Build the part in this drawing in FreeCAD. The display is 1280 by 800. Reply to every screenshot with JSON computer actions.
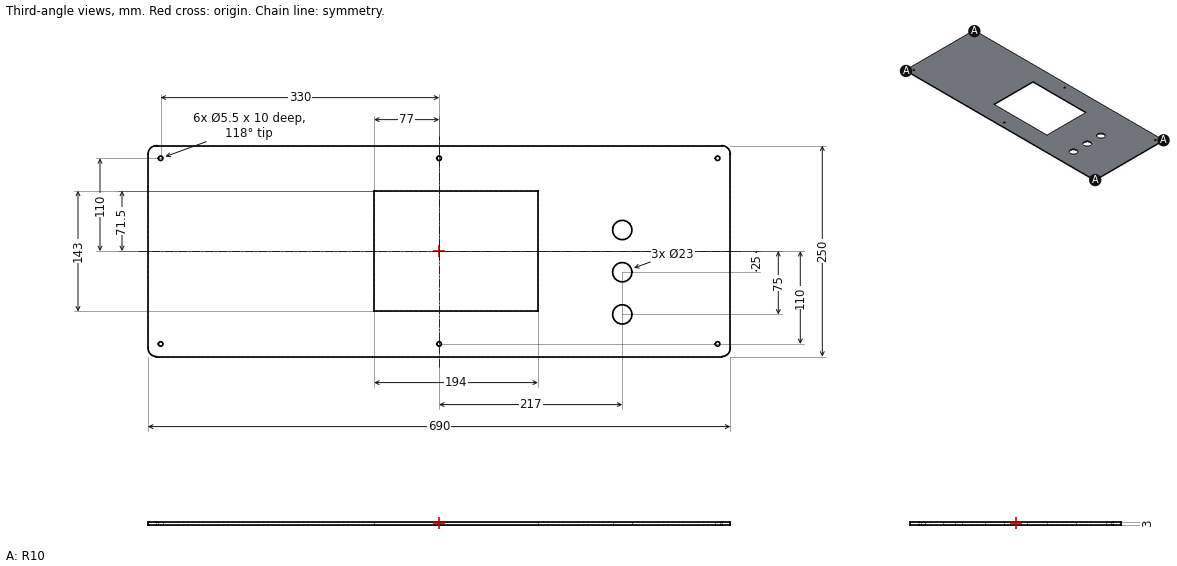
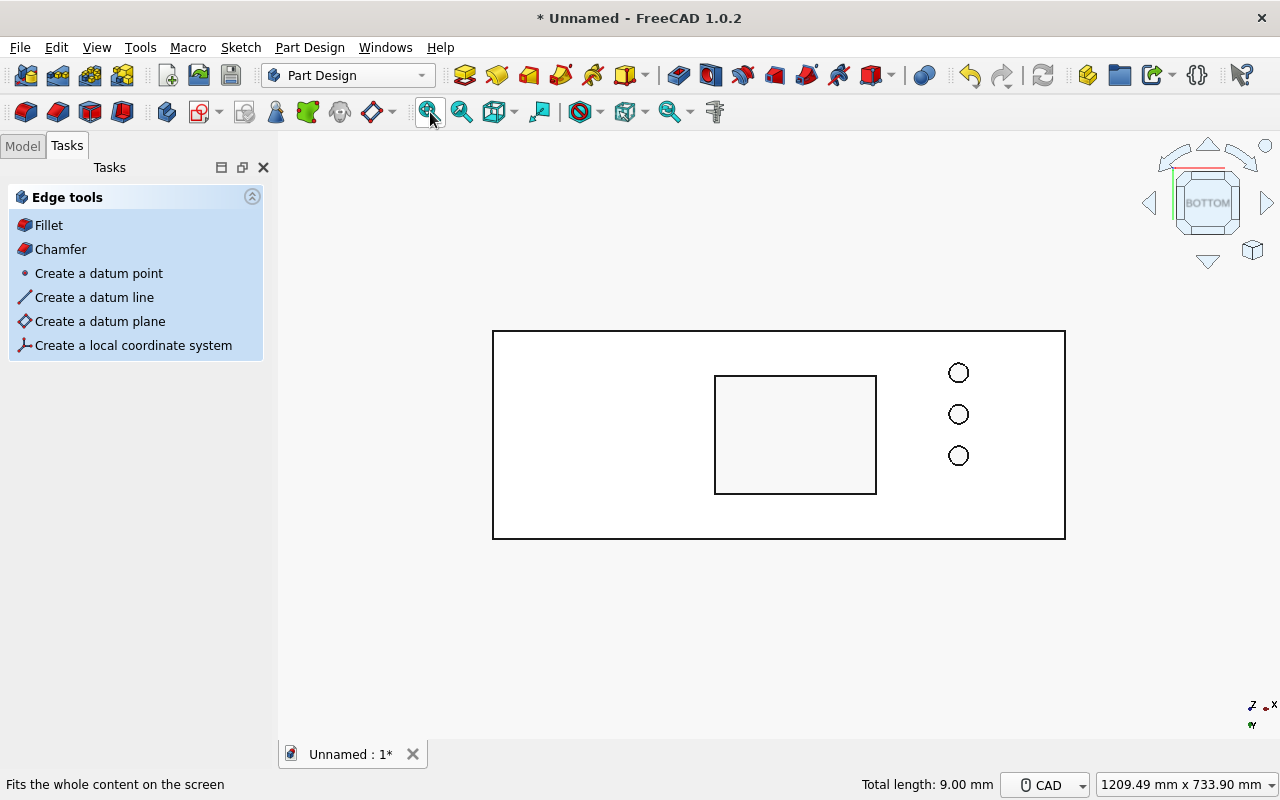
{"action": "scroll", "coordinate": [493, 538], "scroll_direction": "up", "scroll_amount": 14}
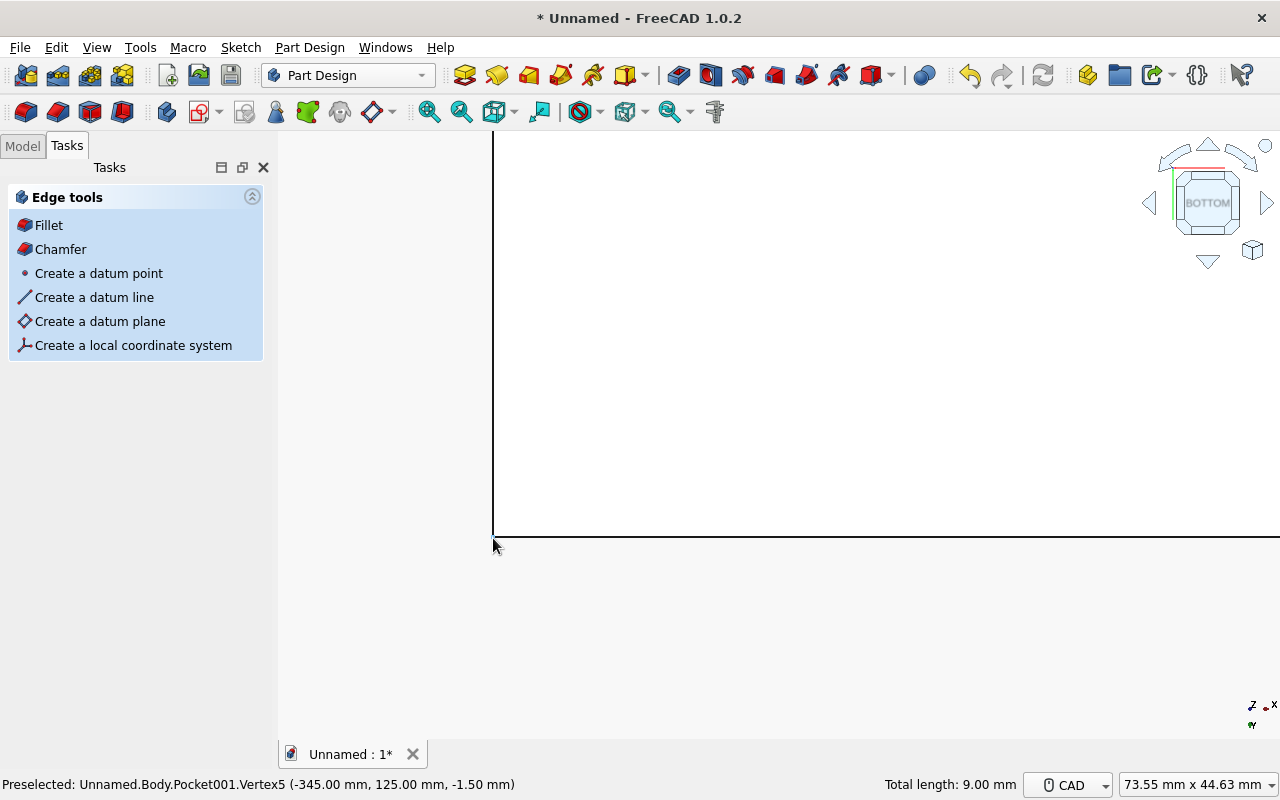
{"action": "left_click", "coordinate": [430, 112]}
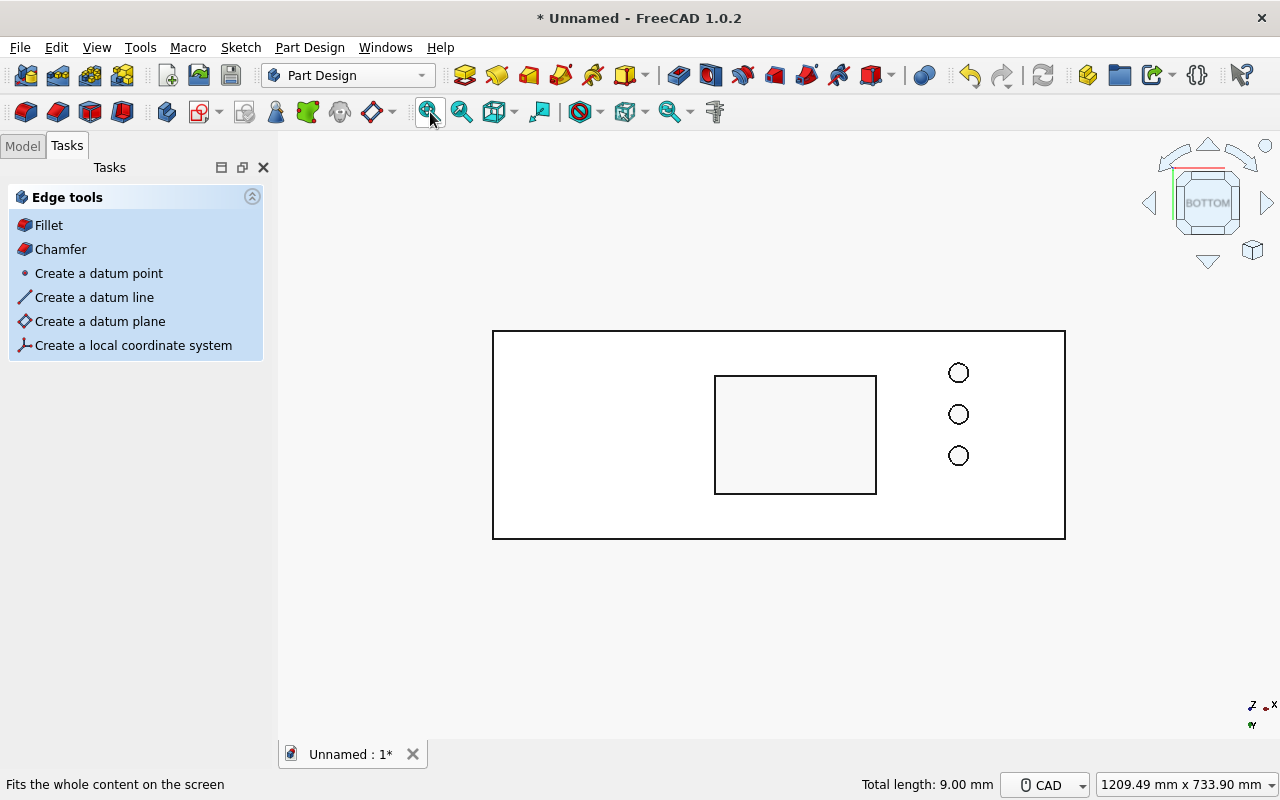
{"action": "key", "text": "4"}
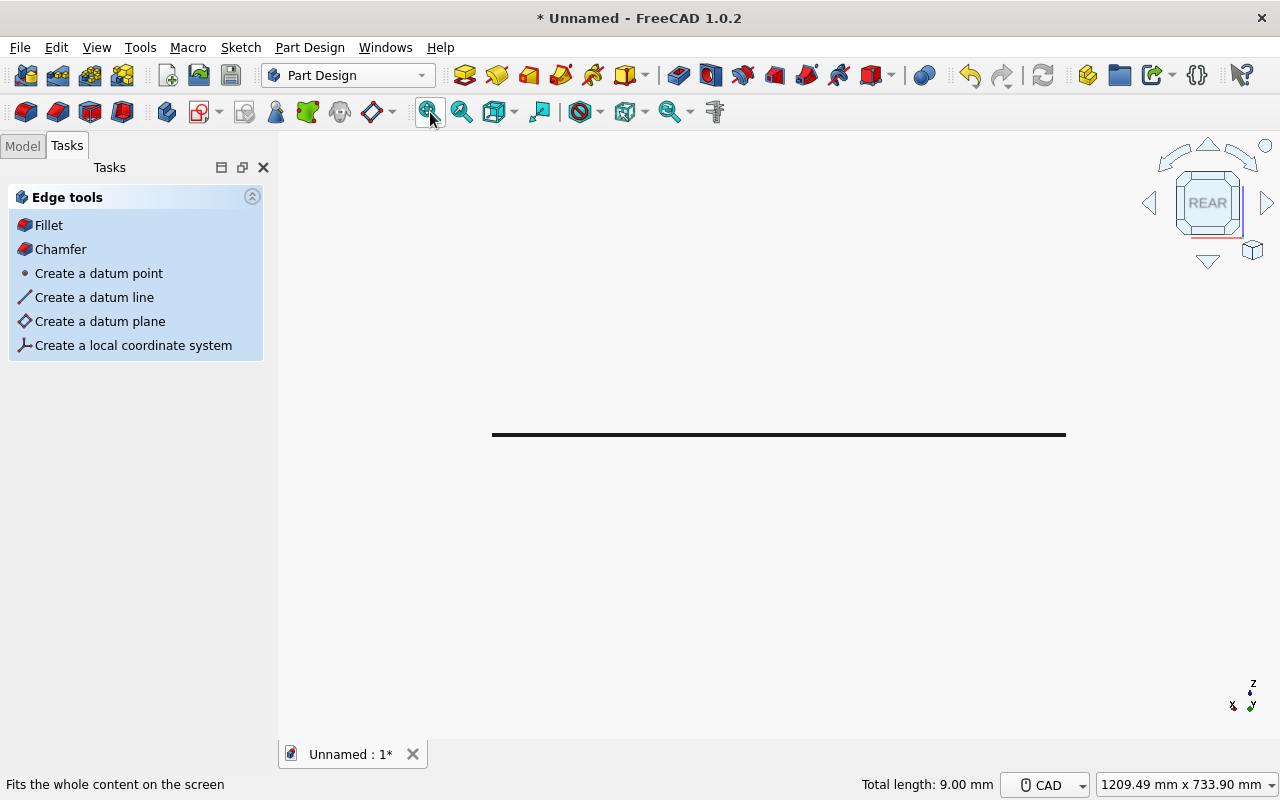
{"action": "scroll", "coordinate": [1065, 434], "scroll_direction": "up", "scroll_amount": 14}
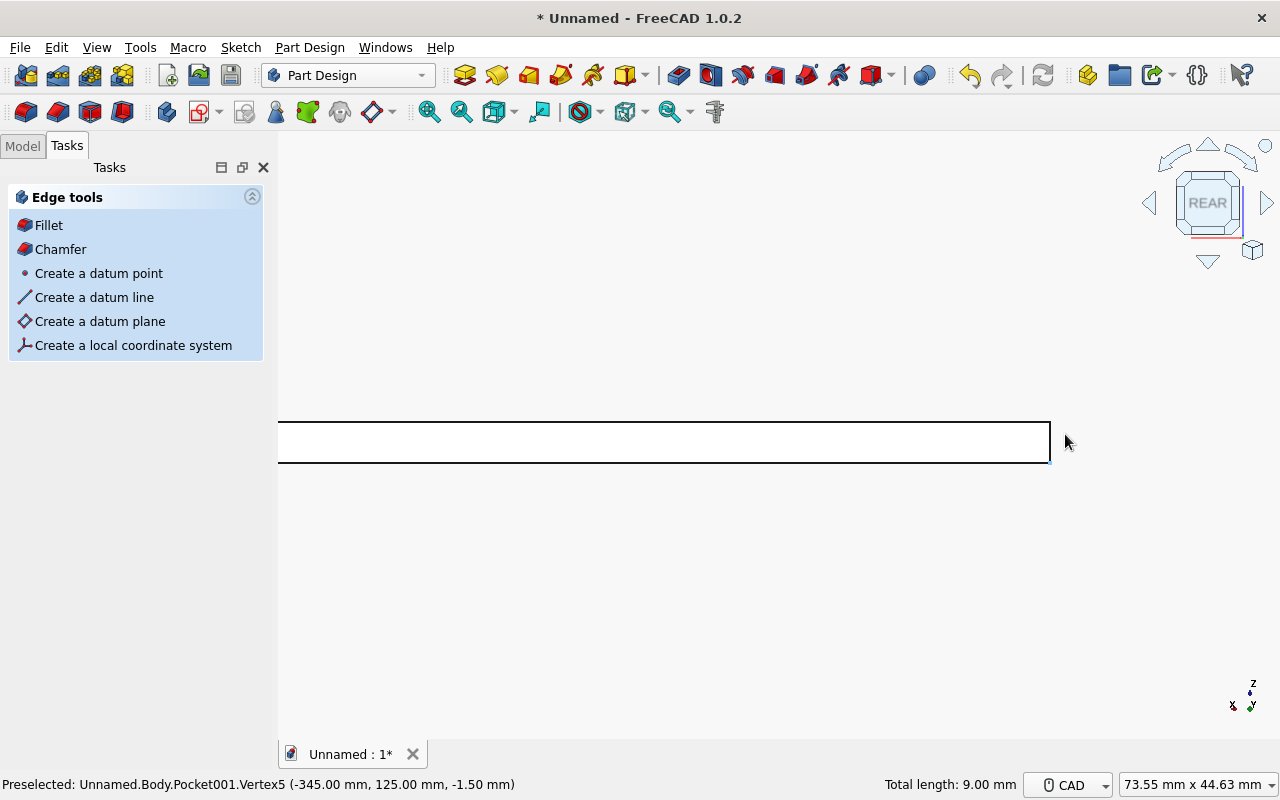
{"action": "left_click", "coordinate": [1050, 442], "text": "ctrl"}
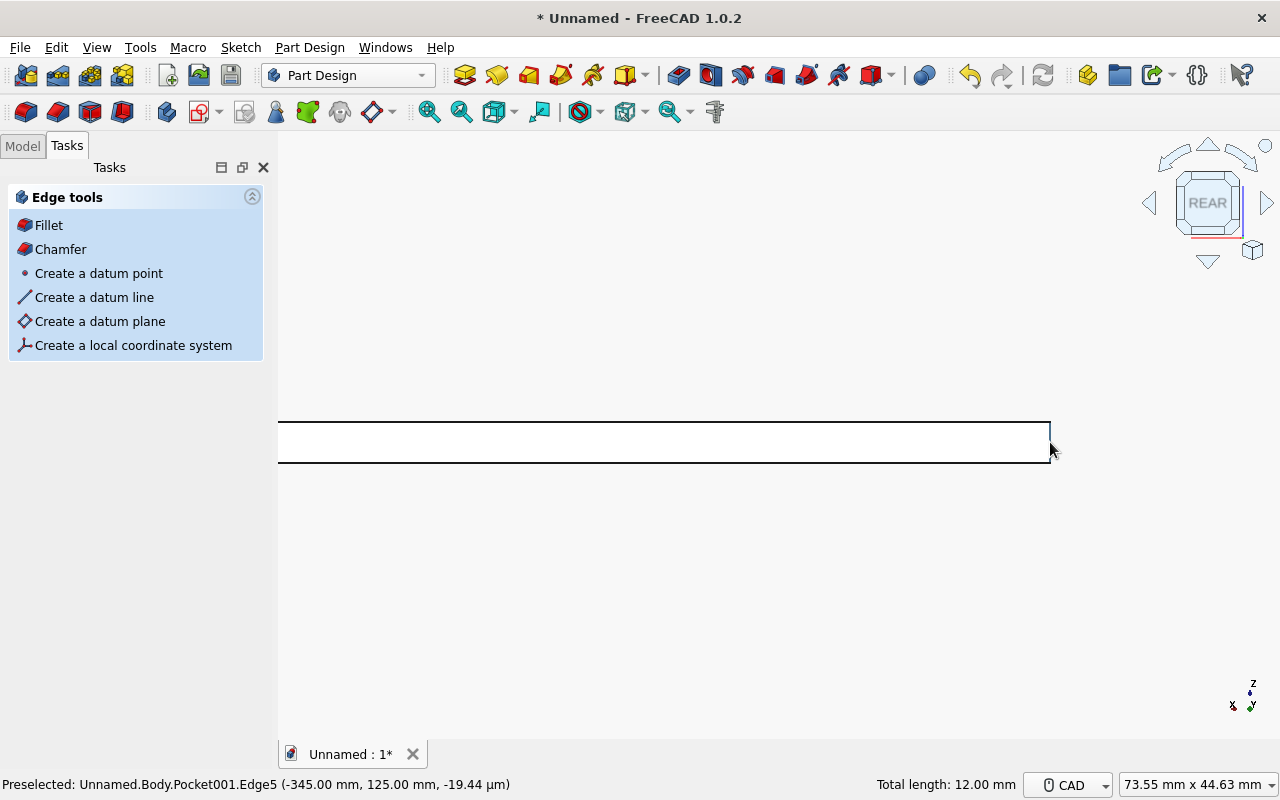
{"action": "left_click", "coordinate": [26, 112]}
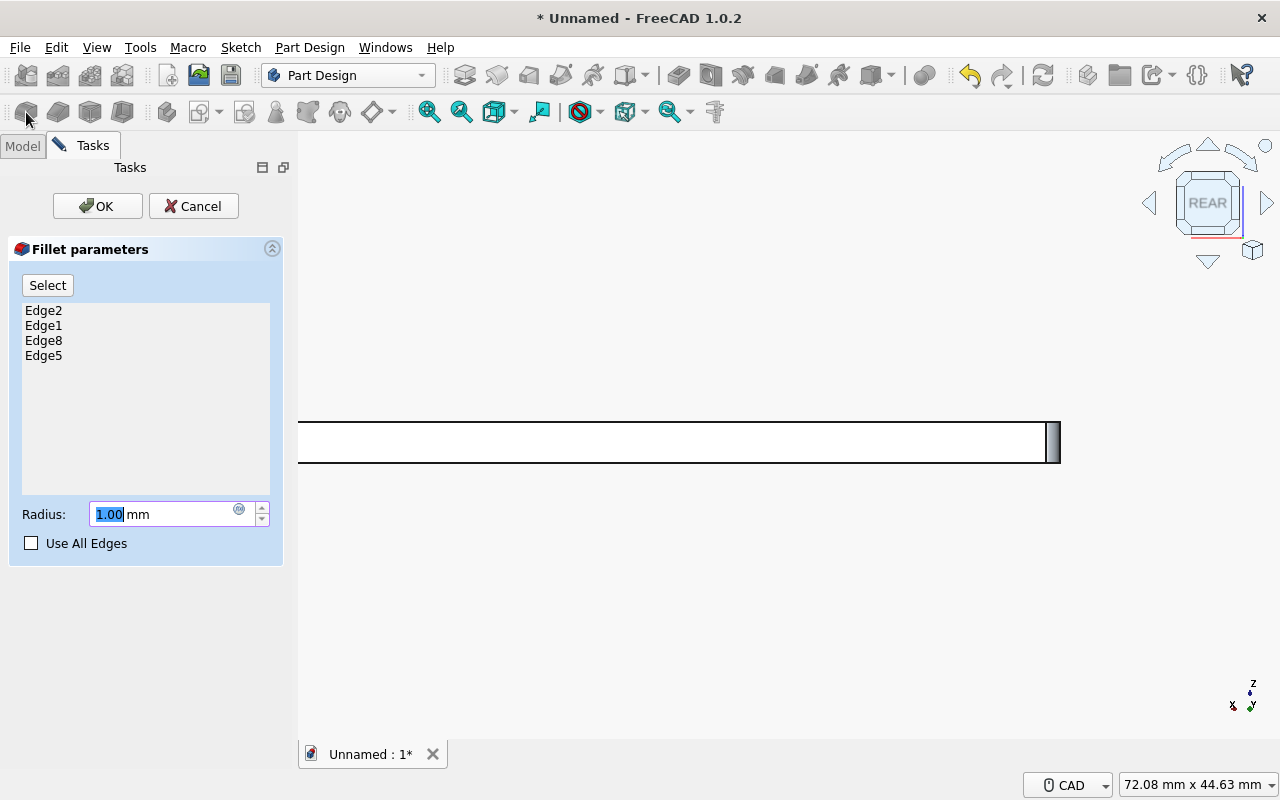
{"action": "type", "text": "10"}
{"action": "key", "text": "Tab"}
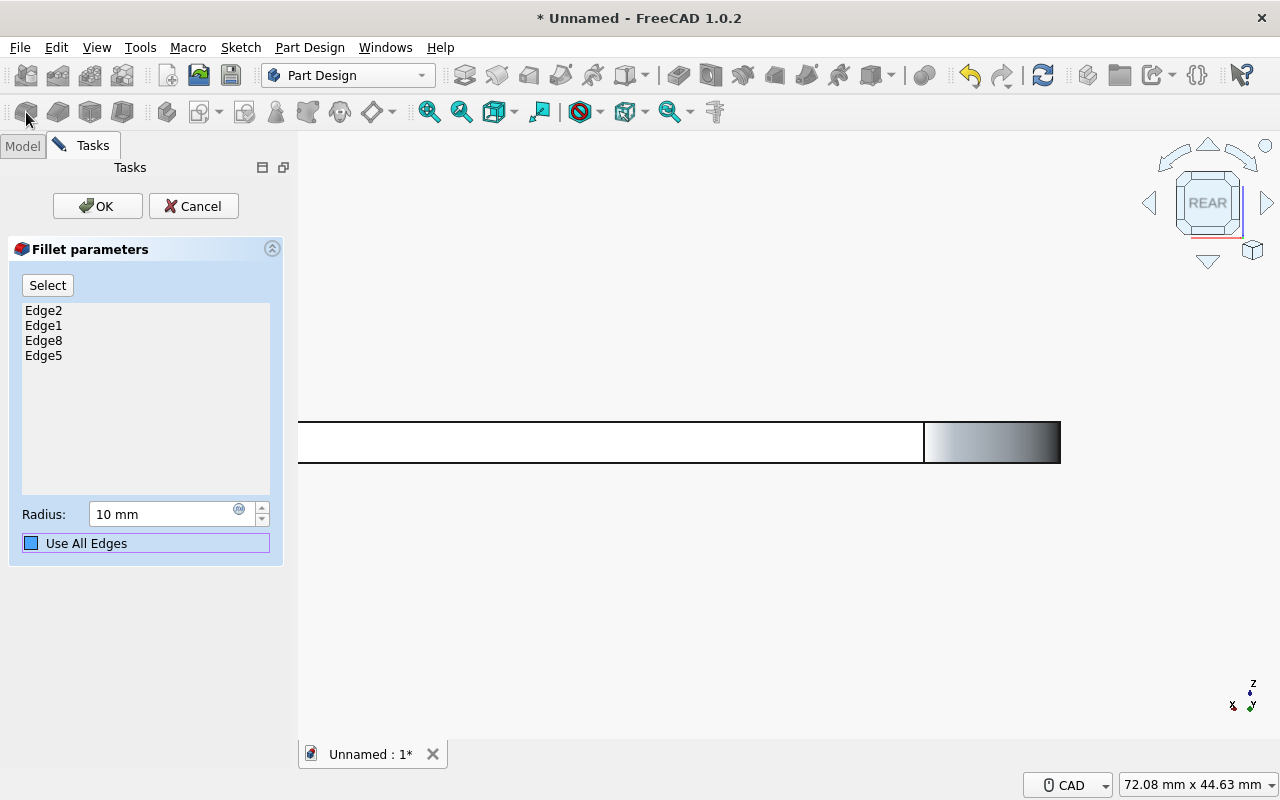
{"action": "left_click", "coordinate": [98, 206]}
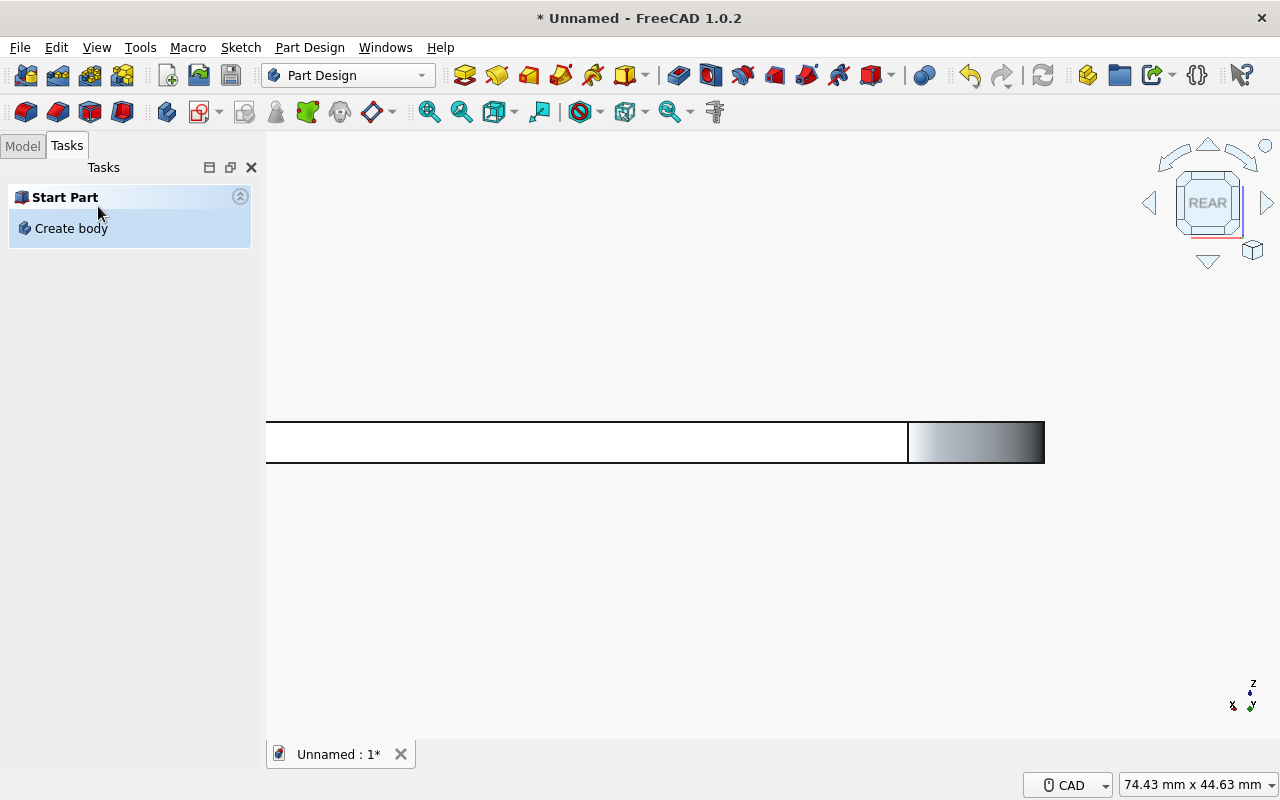
{"action": "left_click", "coordinate": [430, 112]}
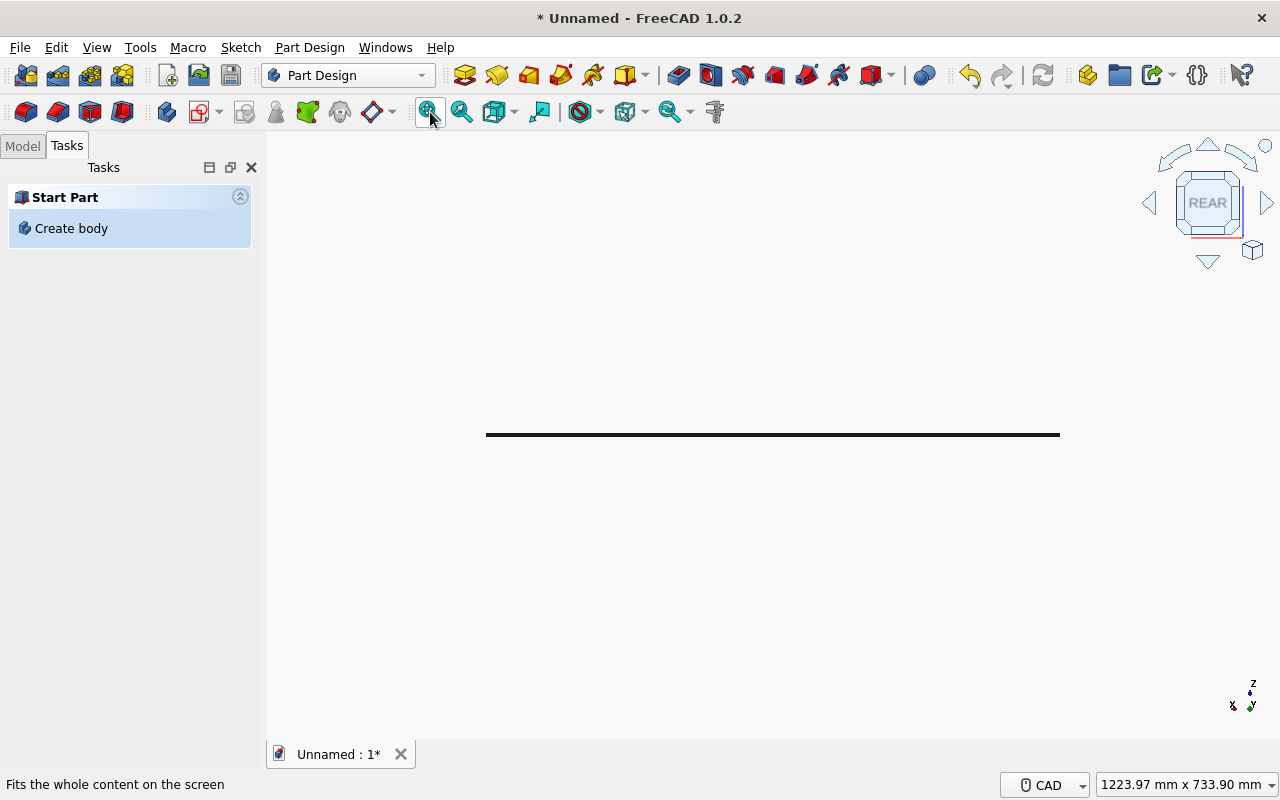
{"action": "key", "text": "0"}